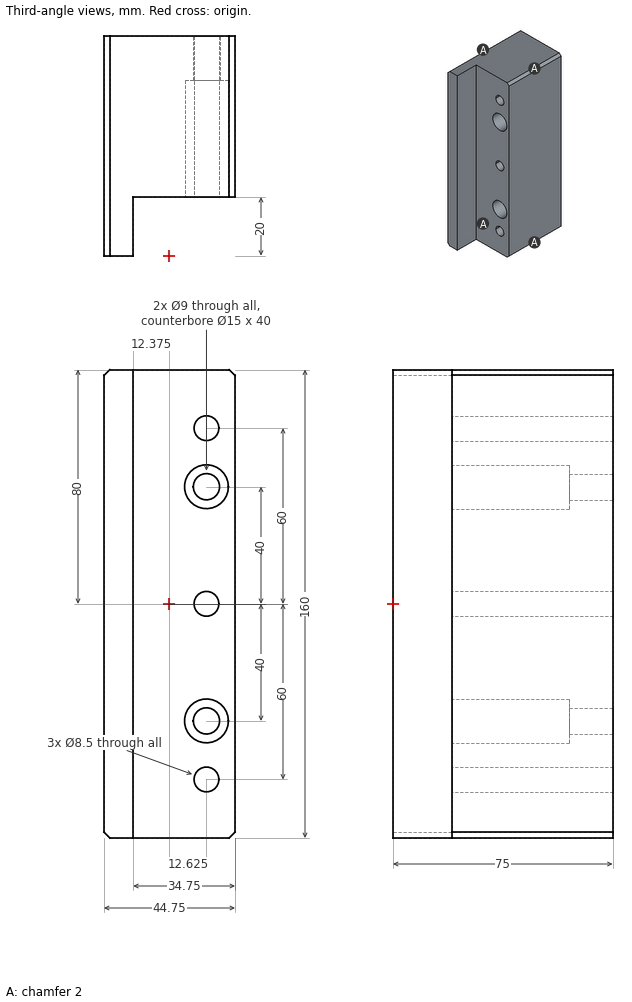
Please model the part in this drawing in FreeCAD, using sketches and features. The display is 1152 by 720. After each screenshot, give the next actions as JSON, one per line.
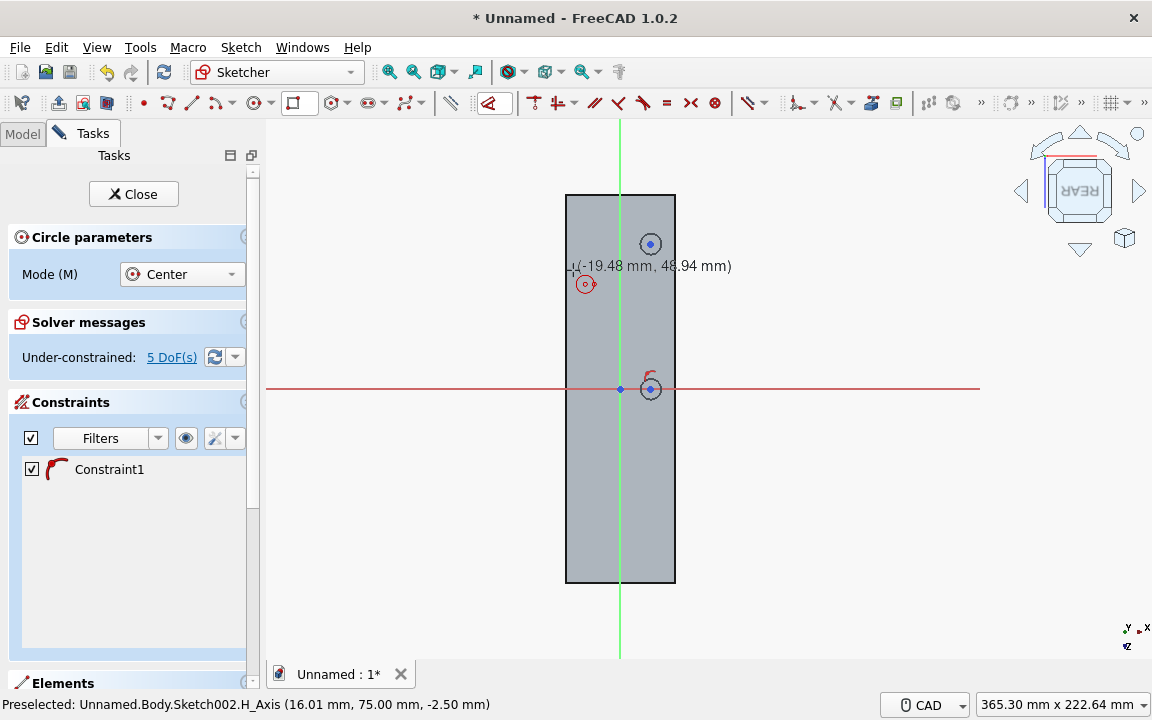
{"action": "scroll", "coordinate": [651, 535], "scroll_direction": "up", "scroll_amount": 4}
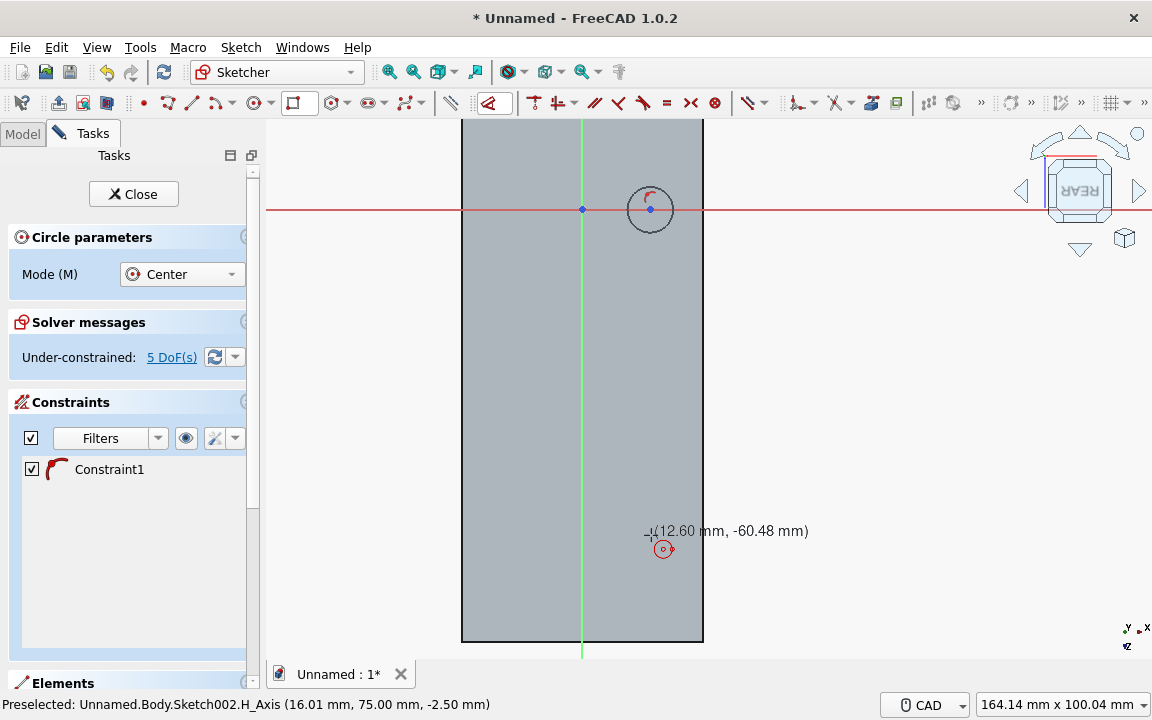
{"action": "left_click", "coordinate": [651, 534]}
{"action": "left_click", "coordinate": [667, 517]}
{"action": "key", "text": "Escape"}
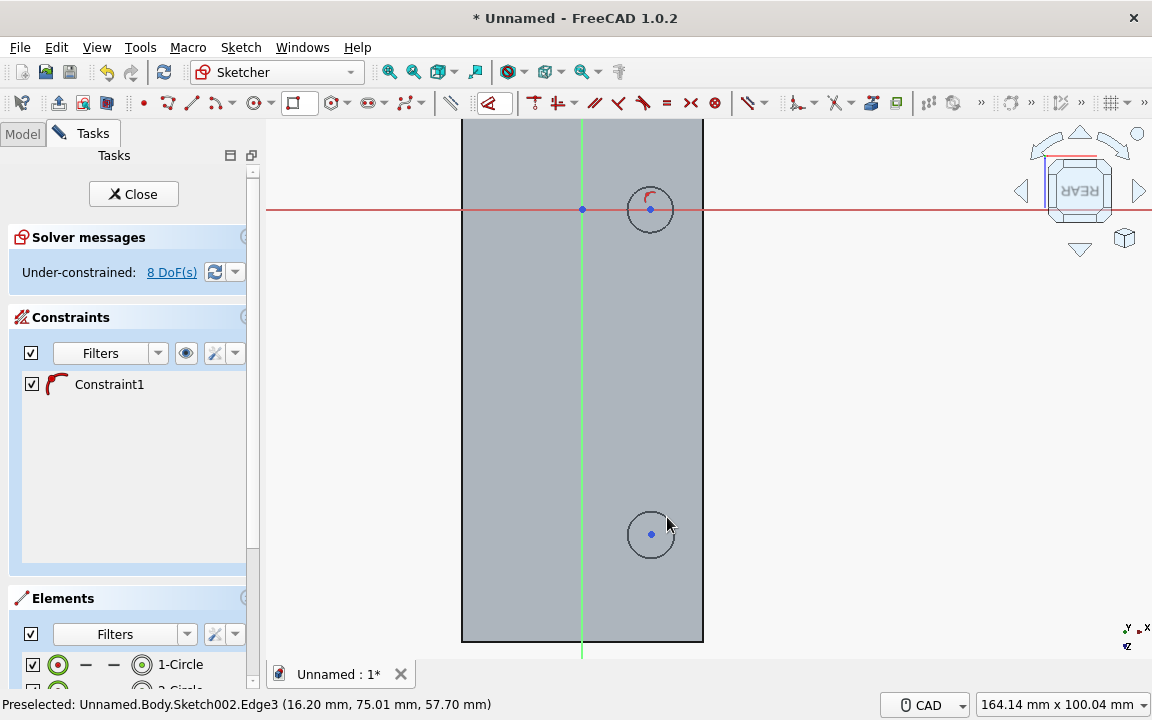
{"action": "scroll", "coordinate": [651, 535], "scroll_direction": "down", "scroll_amount": 4}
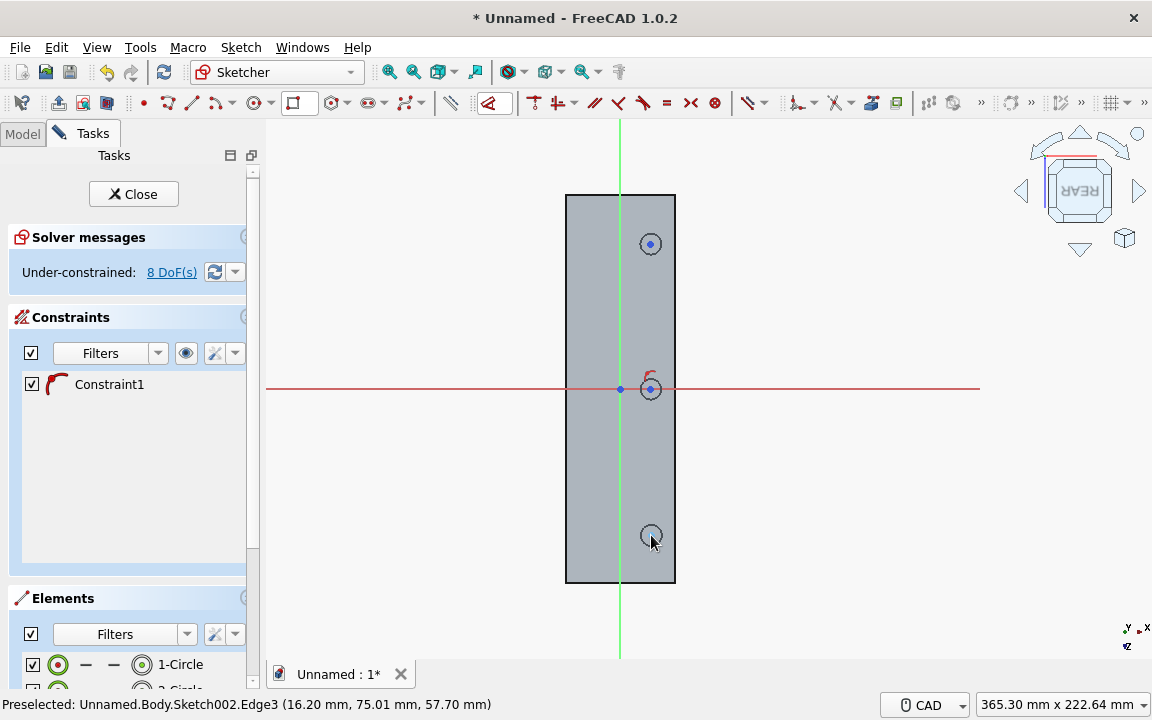
{"action": "scroll", "coordinate": [658, 237], "scroll_direction": "up", "scroll_amount": 2}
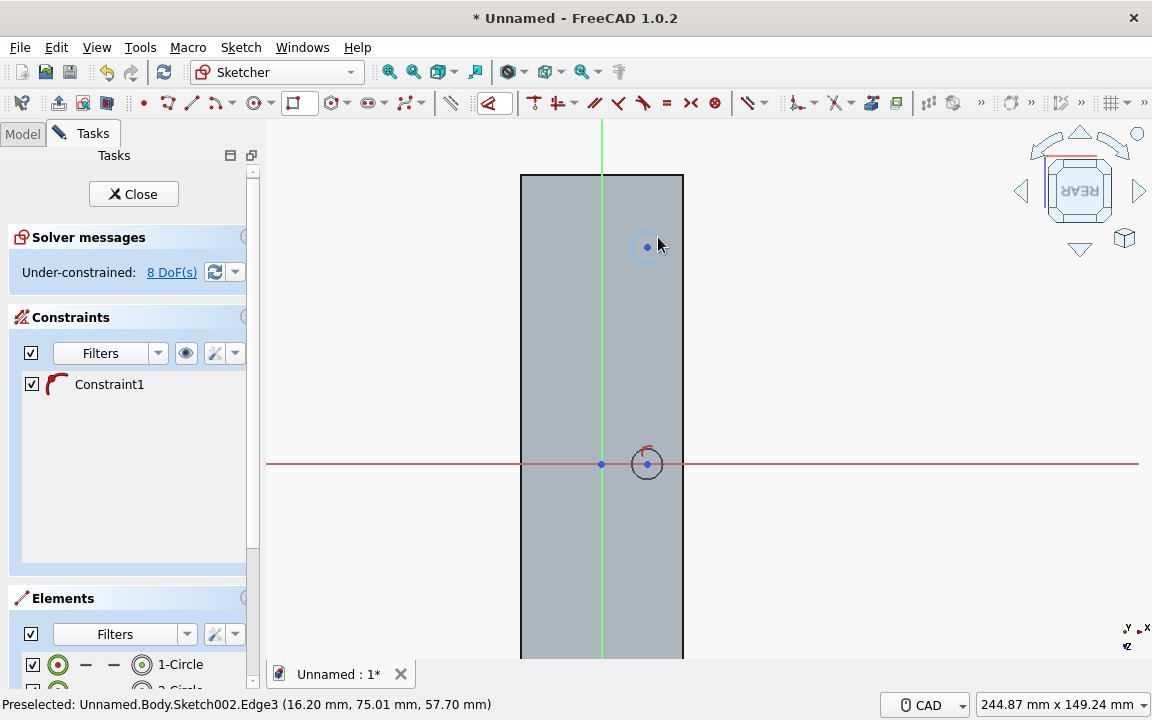
{"action": "left_click", "coordinate": [658, 236]}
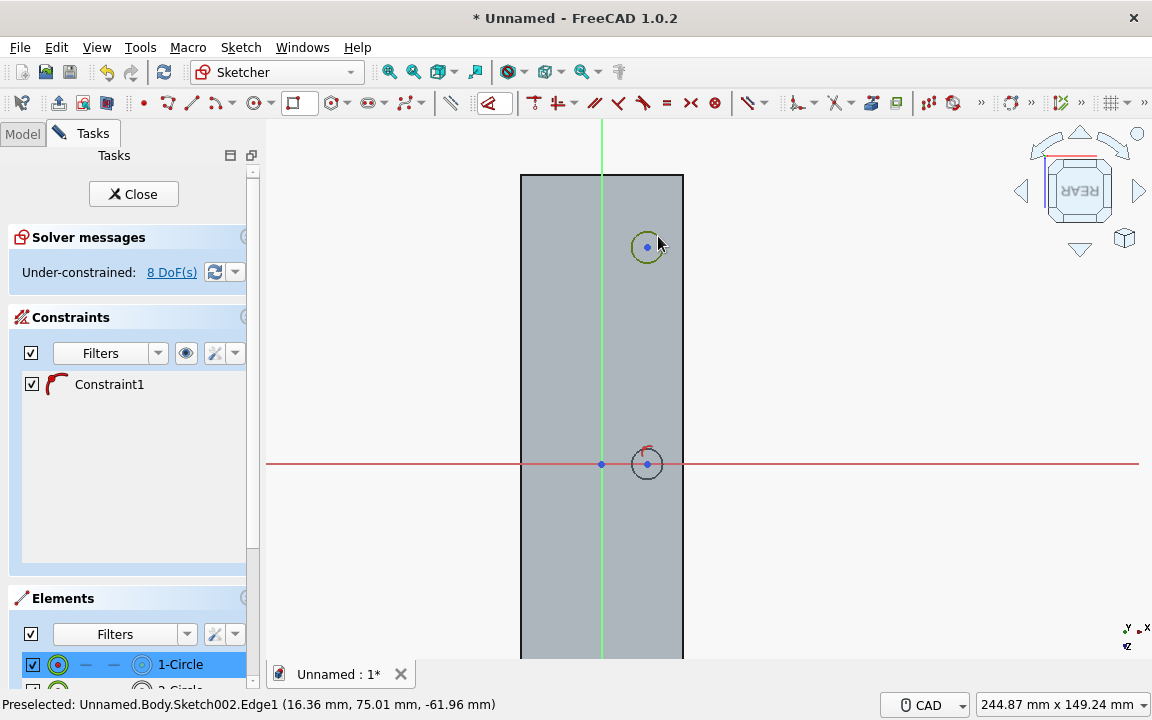
{"action": "scroll", "coordinate": [658, 453], "scroll_direction": "up", "scroll_amount": 2}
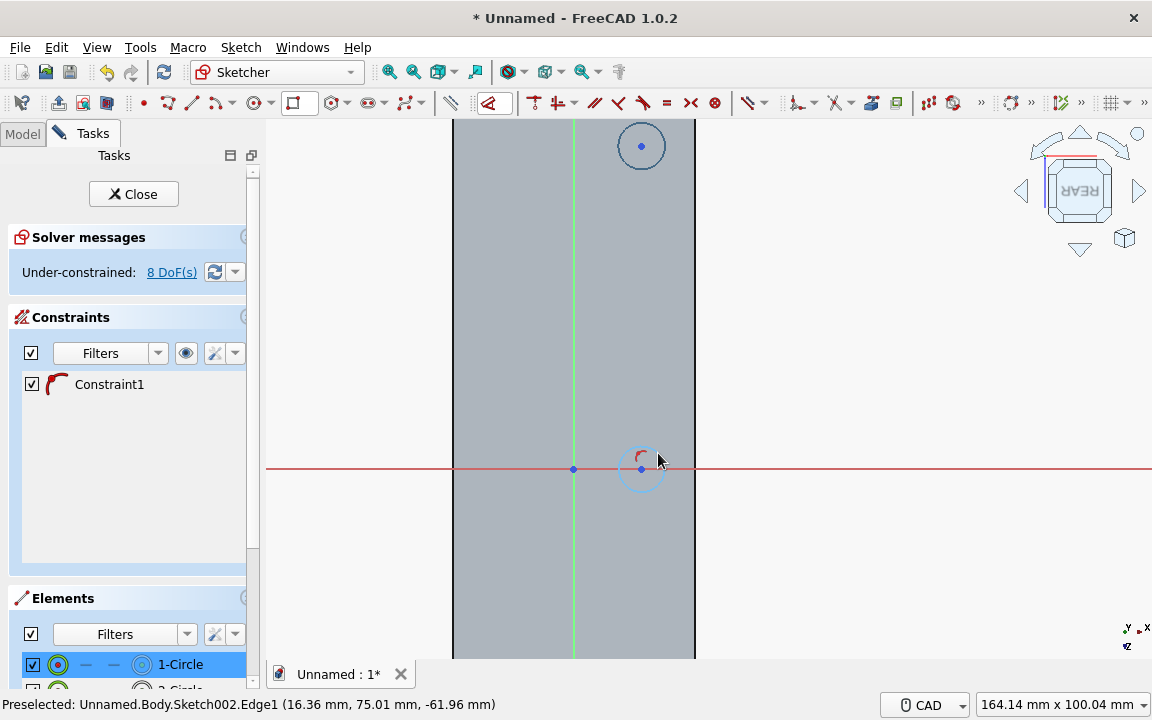
{"action": "left_click", "coordinate": [658, 453]}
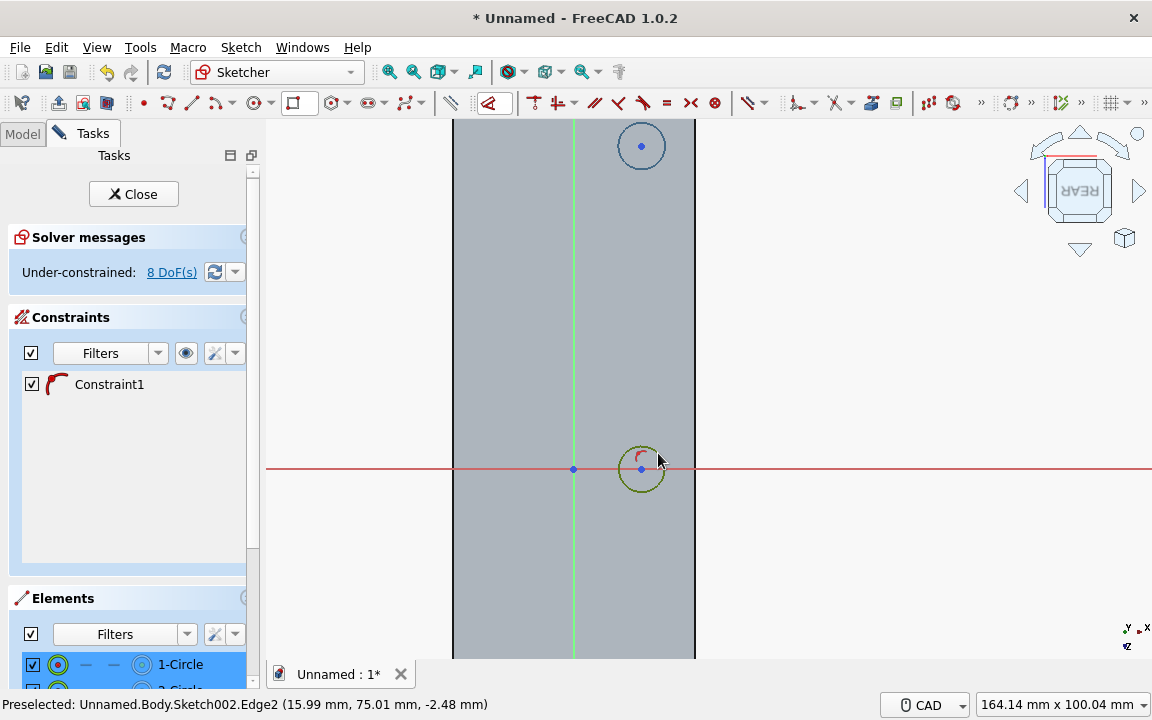
{"action": "scroll", "coordinate": [658, 323], "scroll_direction": "down", "scroll_amount": 4}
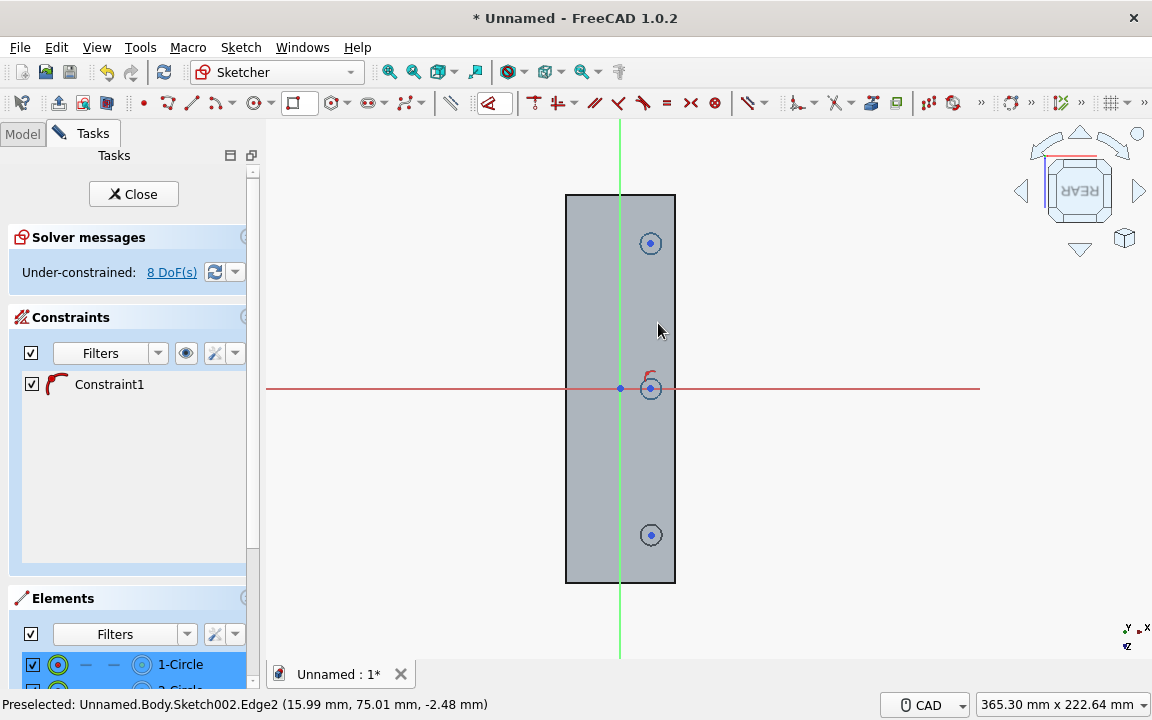
{"action": "scroll", "coordinate": [659, 528], "scroll_direction": "up", "scroll_amount": 2}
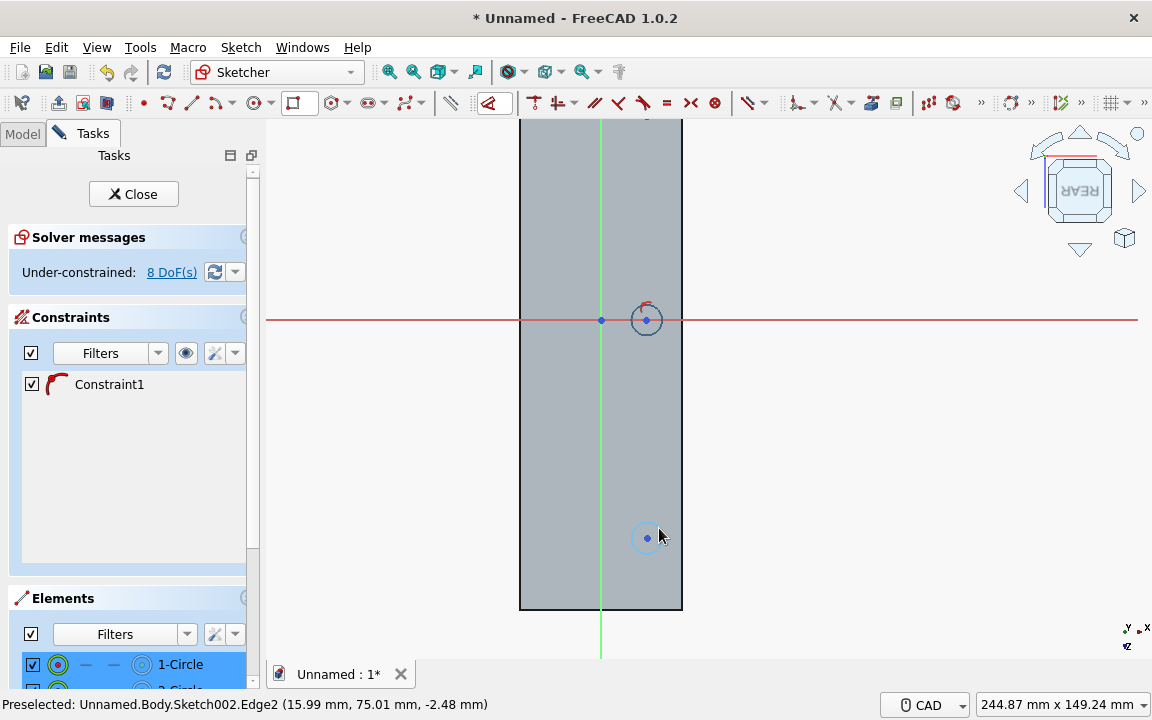
{"action": "left_click", "coordinate": [658, 527]}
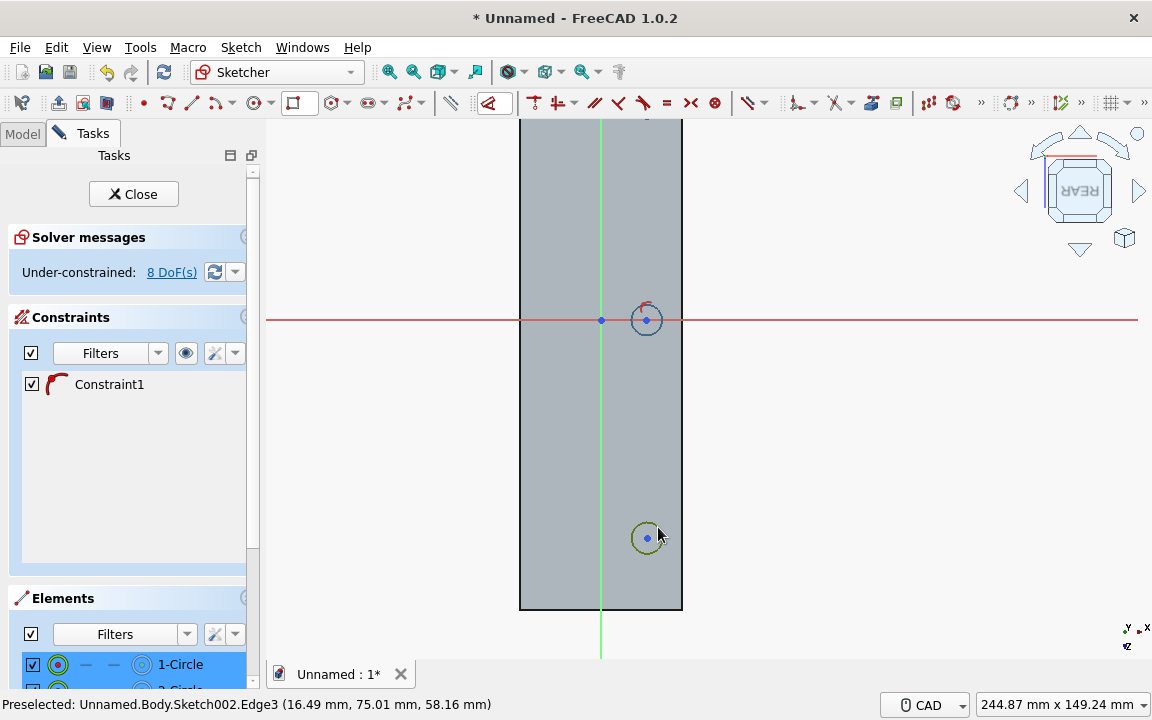
{"action": "left_click", "coordinate": [668, 104]}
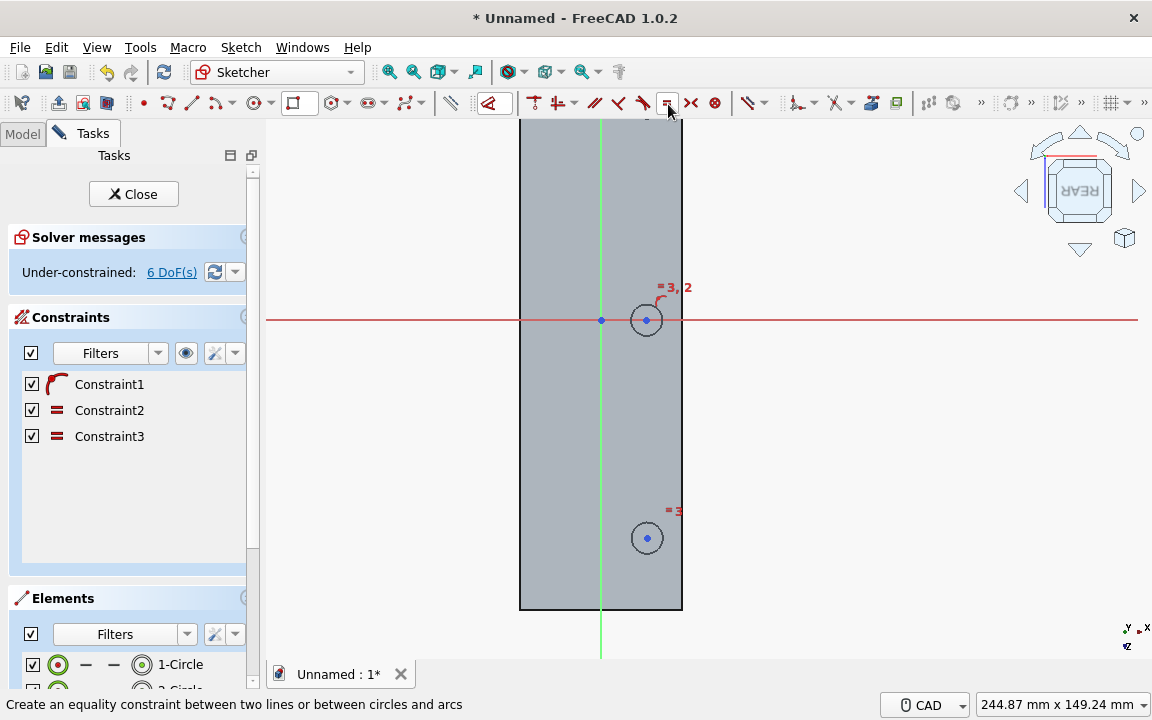
{"action": "scroll", "coordinate": [658, 529], "scroll_direction": "down", "scroll_amount": 2}